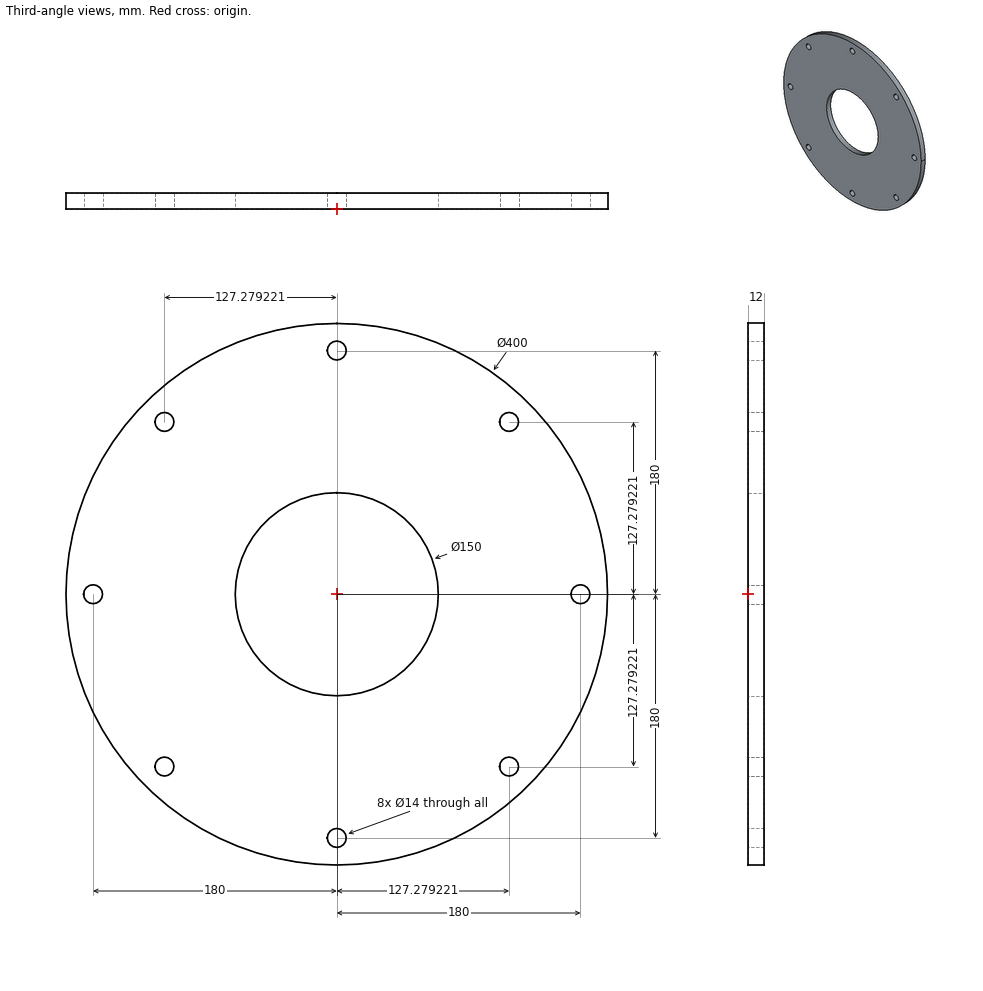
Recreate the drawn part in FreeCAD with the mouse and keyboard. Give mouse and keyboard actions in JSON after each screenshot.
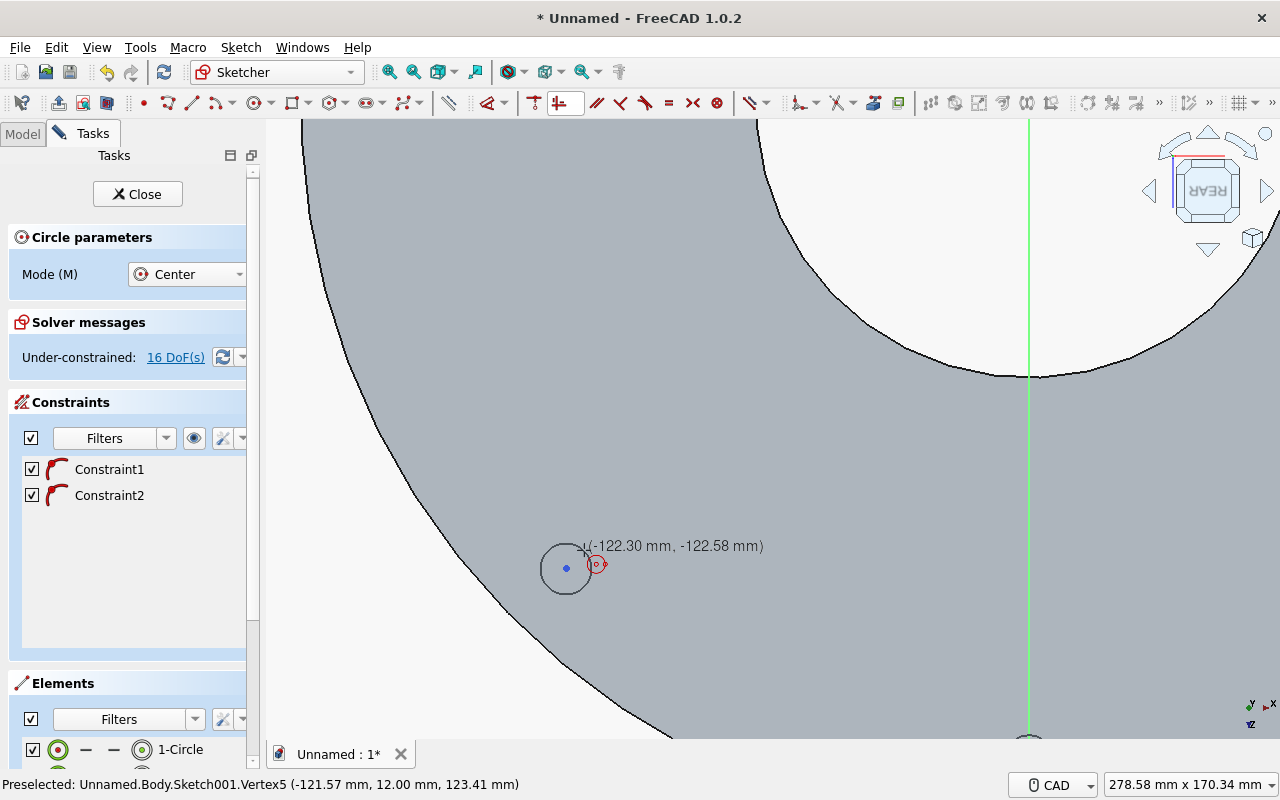
{"action": "scroll", "coordinate": [565, 569], "scroll_direction": "down", "scroll_amount": 6}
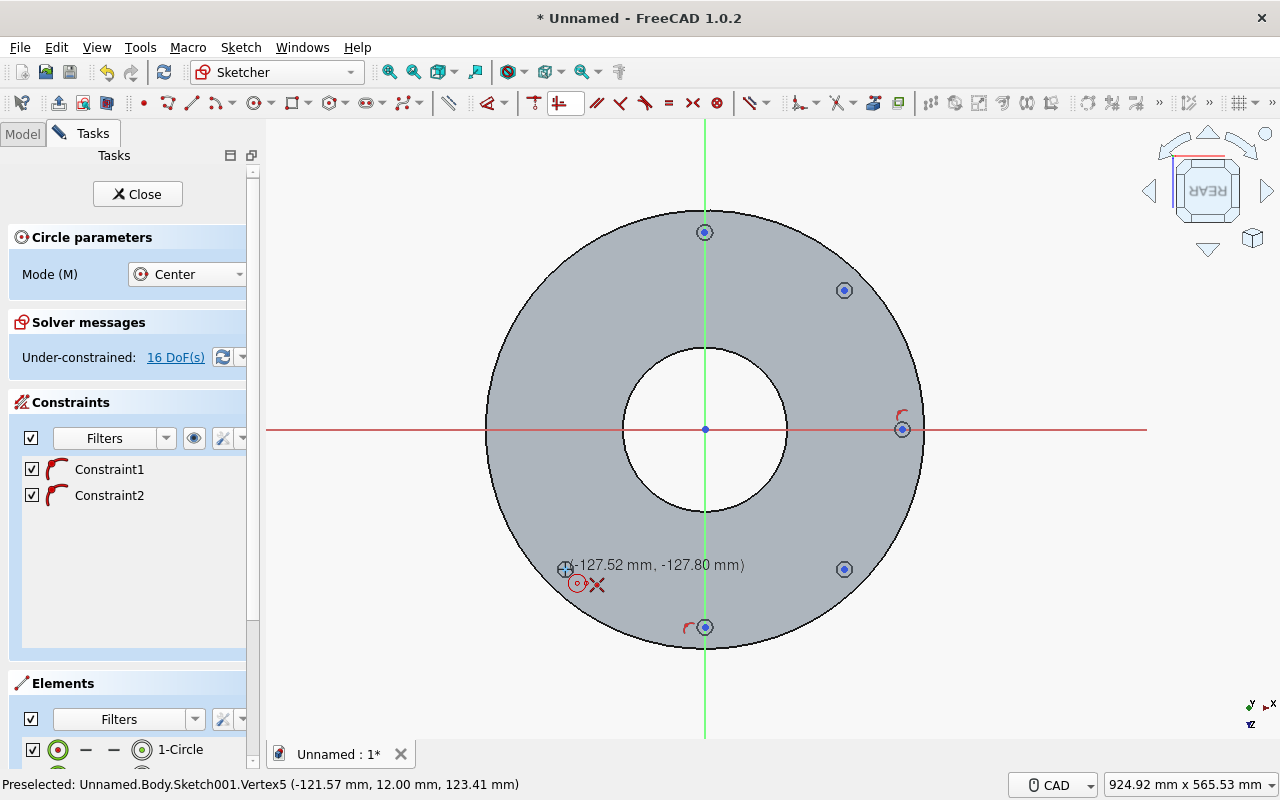
{"action": "scroll", "coordinate": [508, 430], "scroll_direction": "up", "scroll_amount": 6}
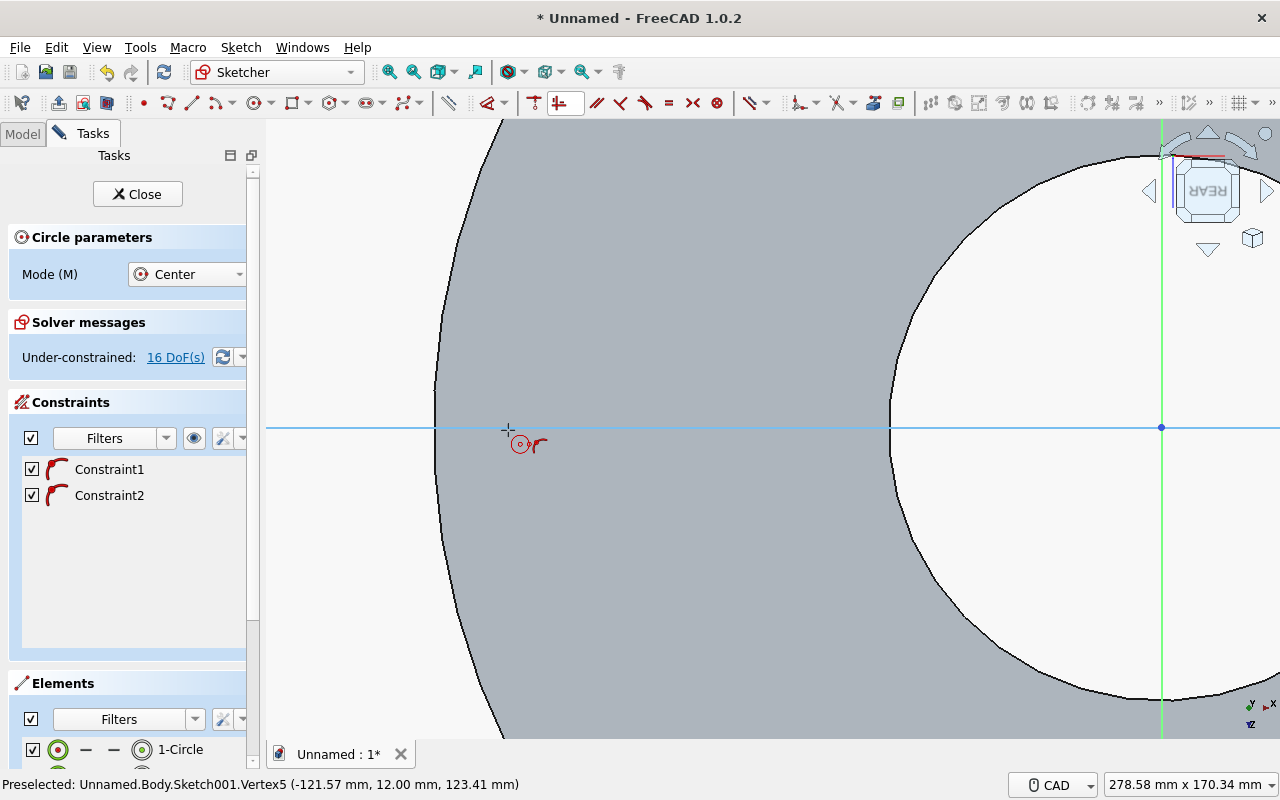
{"action": "left_click", "coordinate": [506, 428]}
{"action": "left_click", "coordinate": [524, 410]}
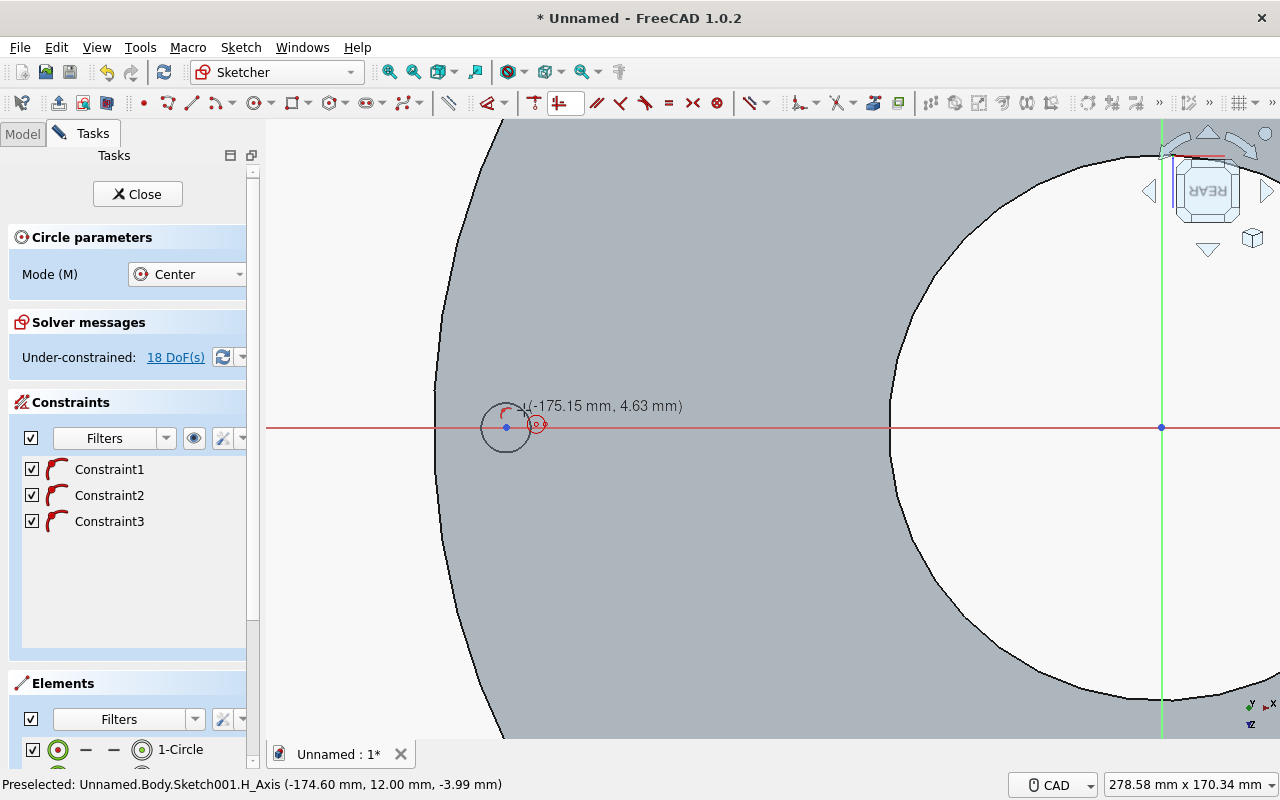
{"action": "scroll", "coordinate": [508, 430], "scroll_direction": "down", "scroll_amount": 6}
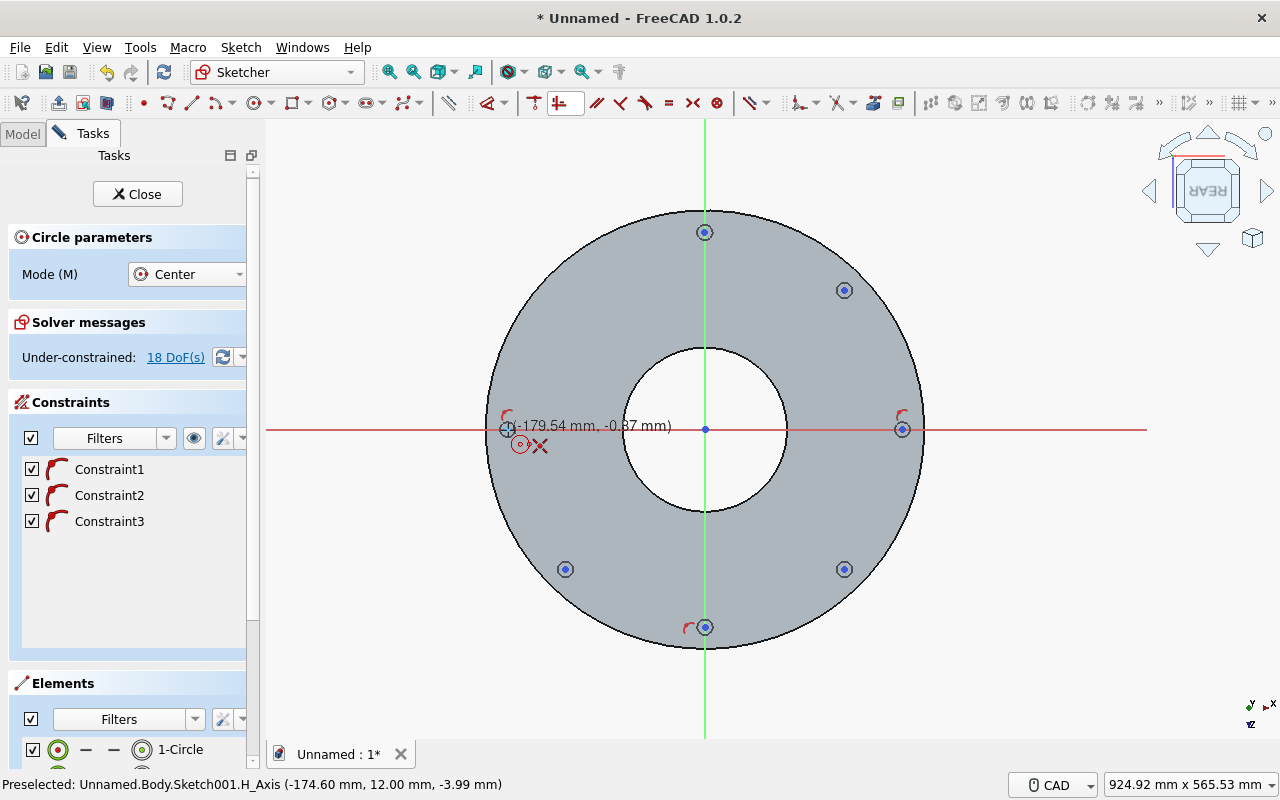
{"action": "scroll", "coordinate": [565, 290], "scroll_direction": "up", "scroll_amount": 6}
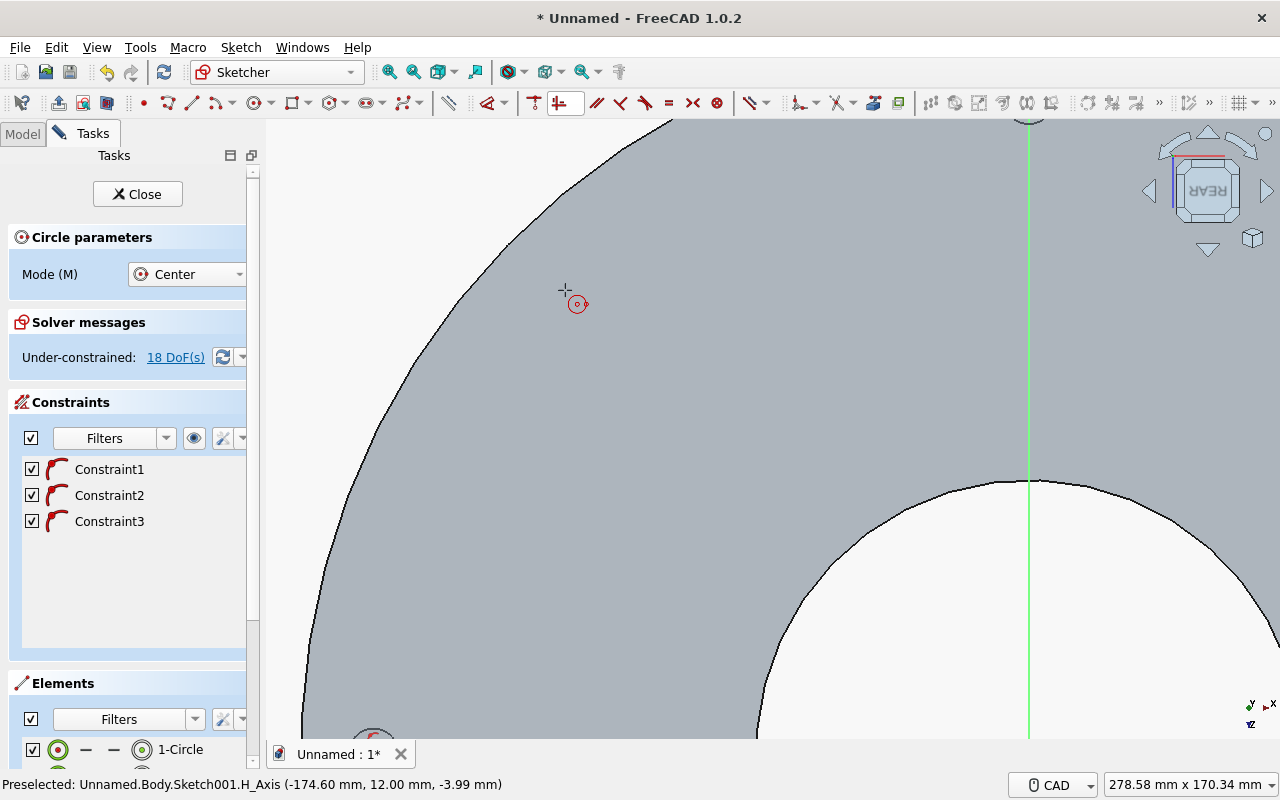
{"action": "left_click", "coordinate": [566, 290]}
{"action": "left_click", "coordinate": [584, 272]}
{"action": "key", "text": "Escape"}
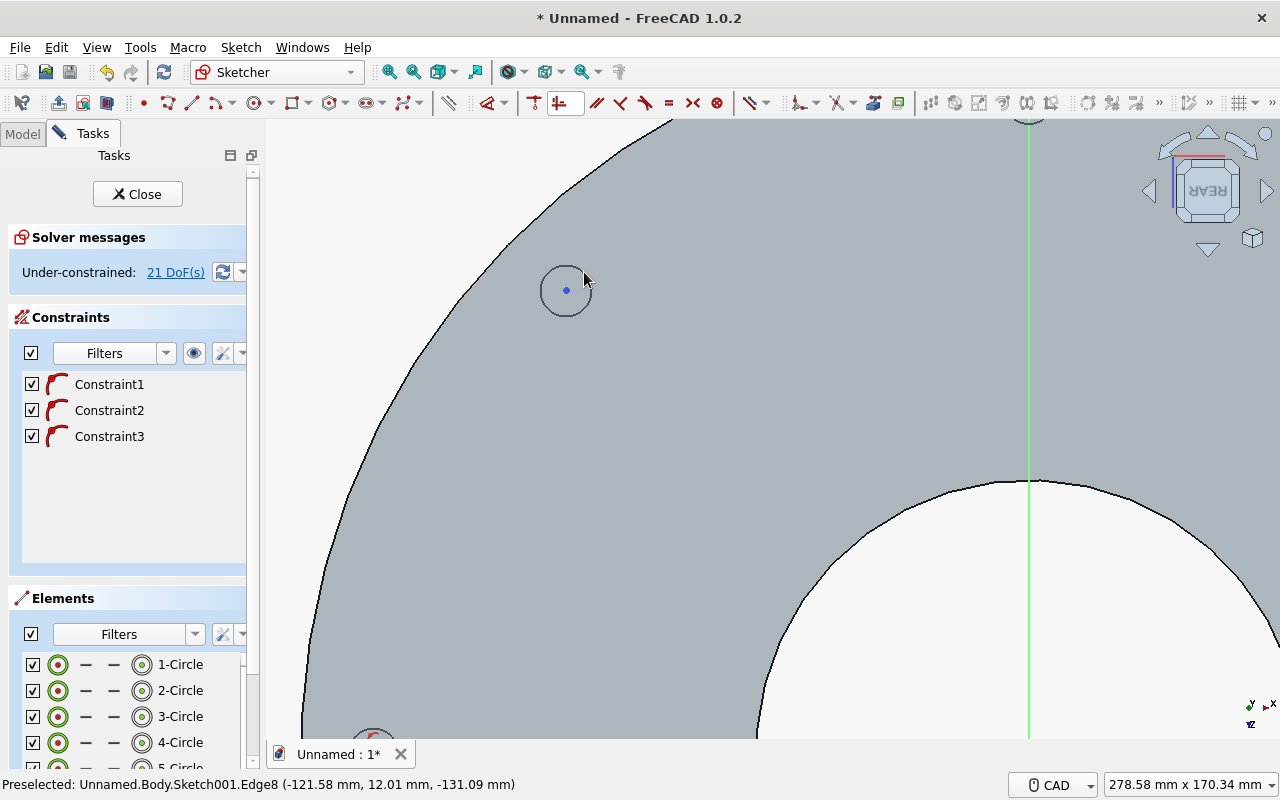
{"action": "scroll", "coordinate": [565, 289], "scroll_direction": "down", "scroll_amount": 6}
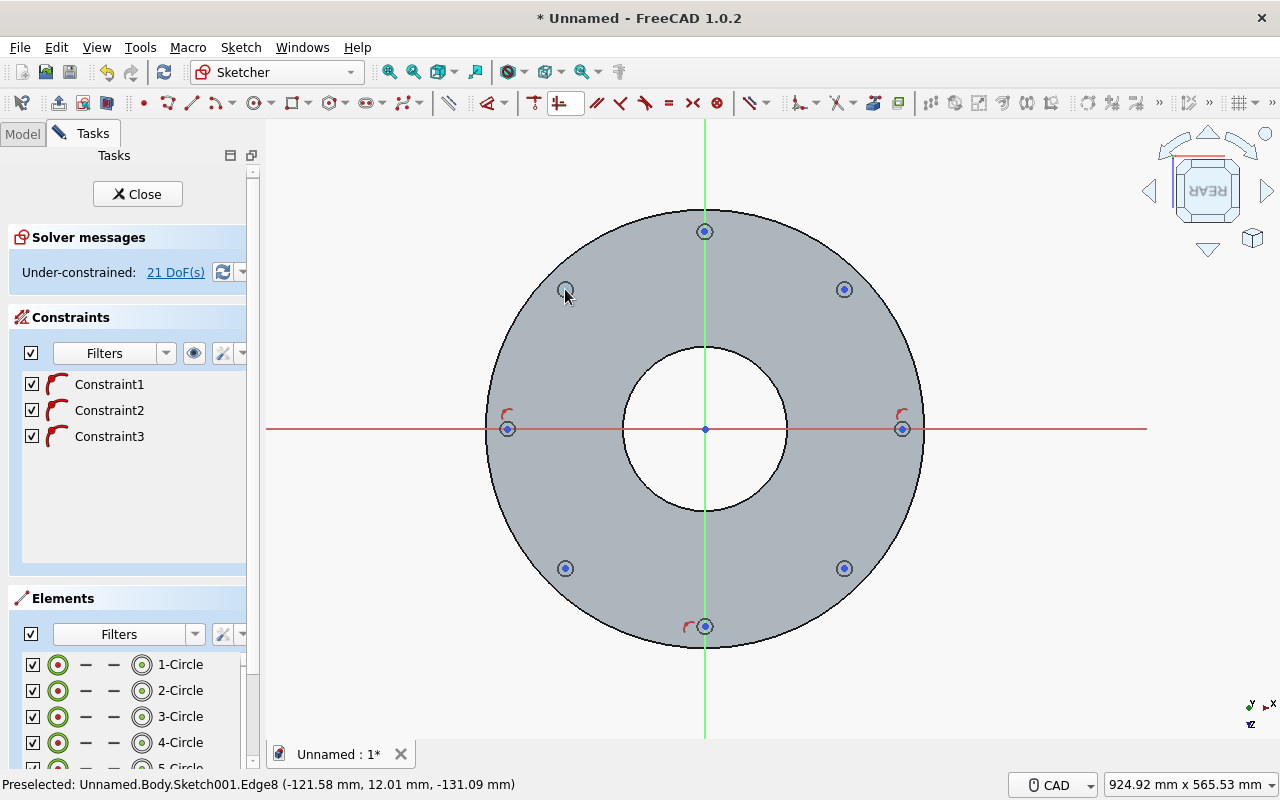
{"action": "scroll", "coordinate": [710, 226], "scroll_direction": "up", "scroll_amount": 5}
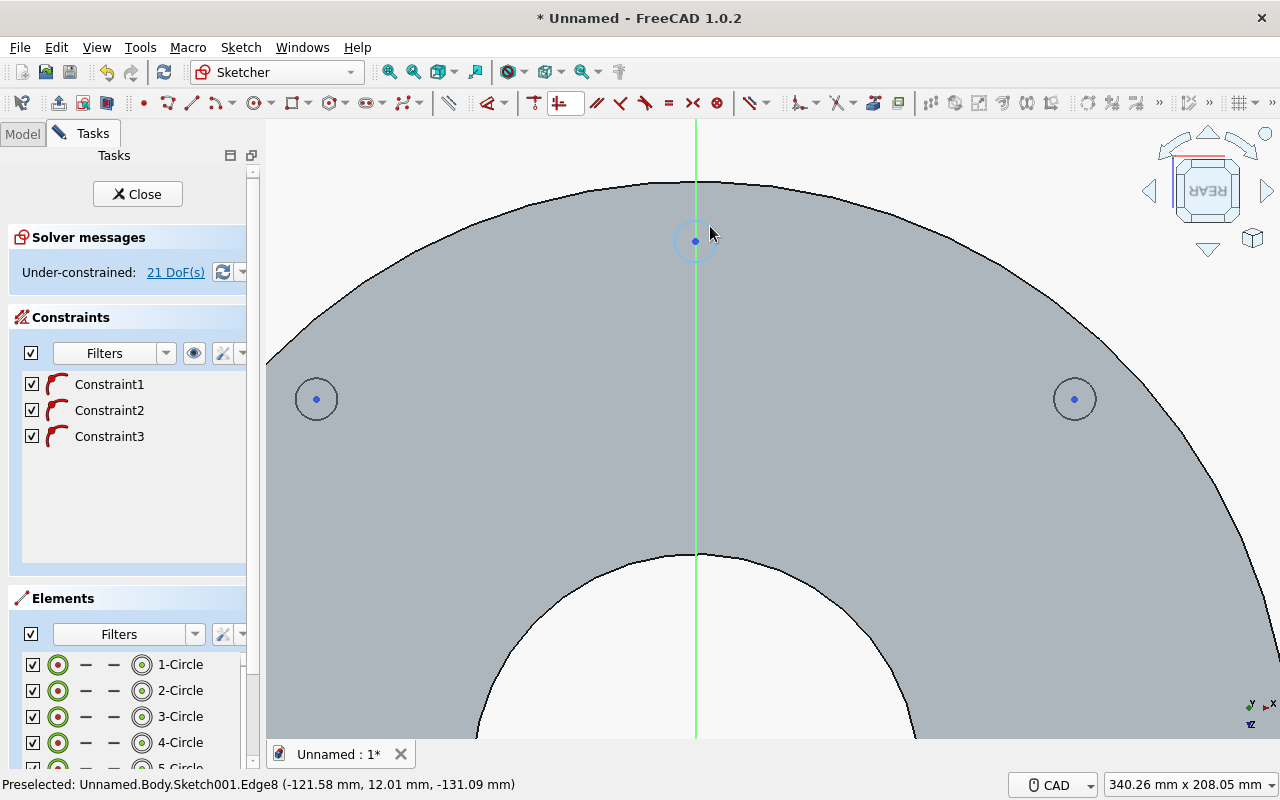
{"action": "left_click", "coordinate": [710, 227]}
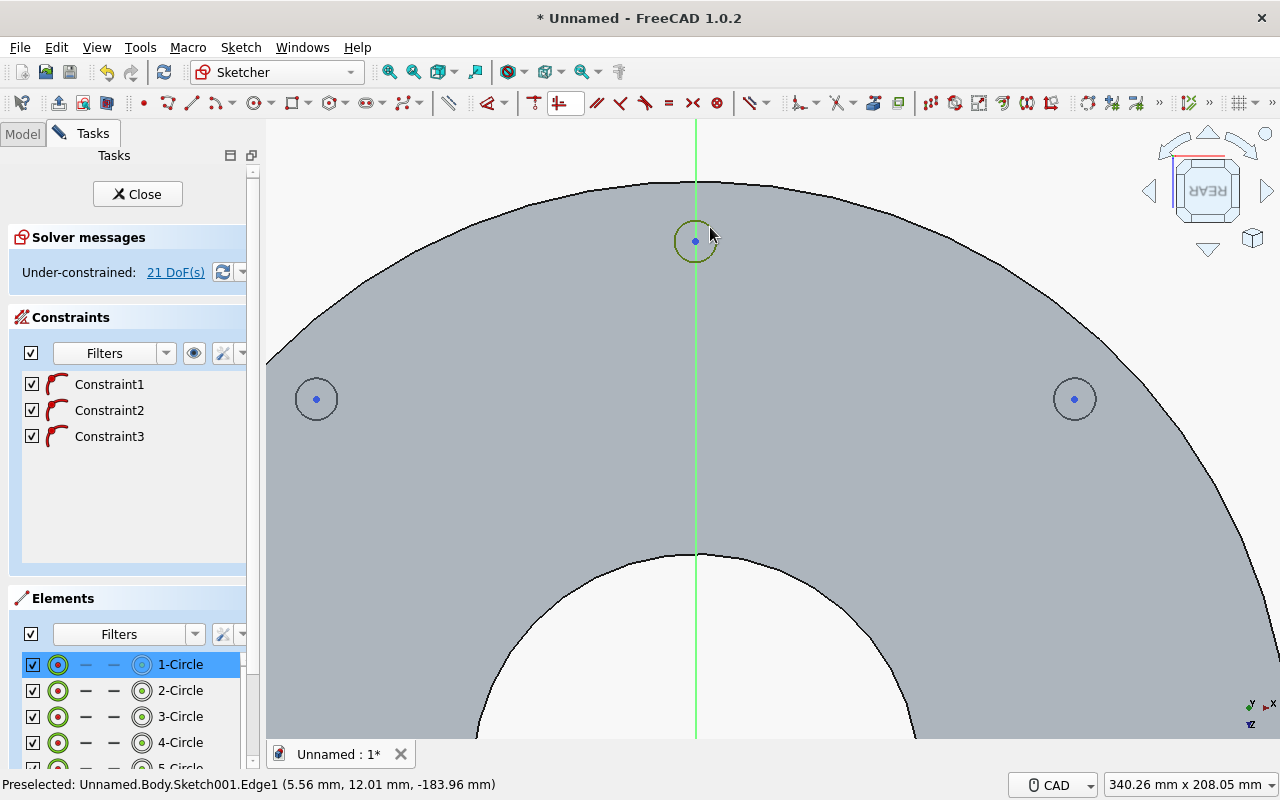
{"action": "left_click", "coordinate": [1090, 384]}